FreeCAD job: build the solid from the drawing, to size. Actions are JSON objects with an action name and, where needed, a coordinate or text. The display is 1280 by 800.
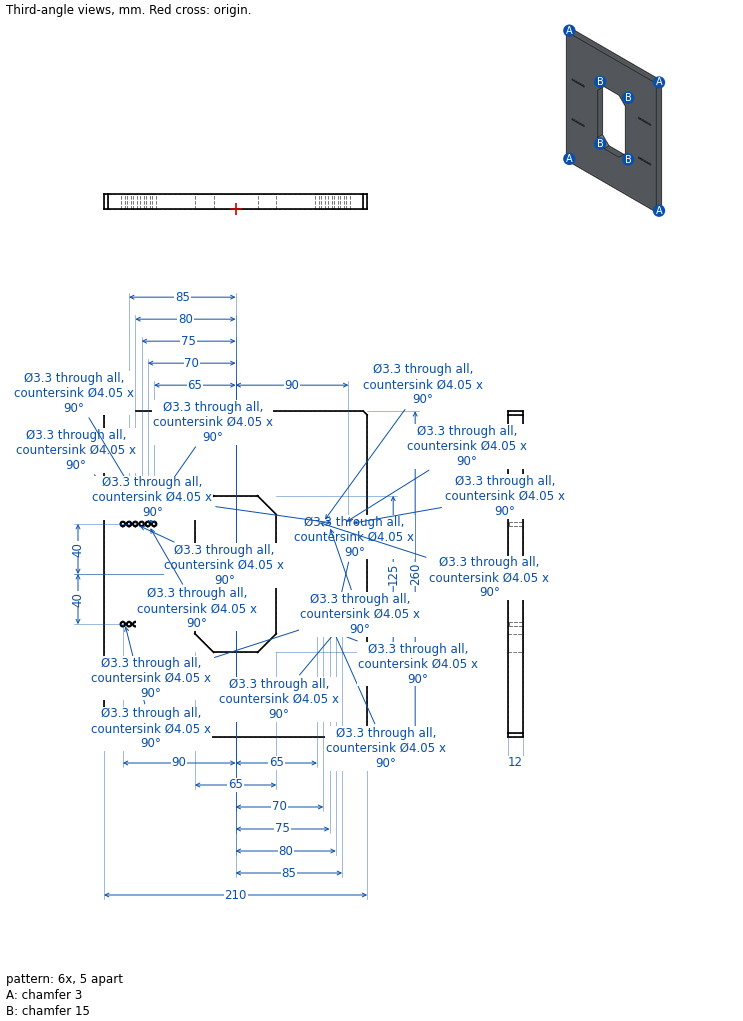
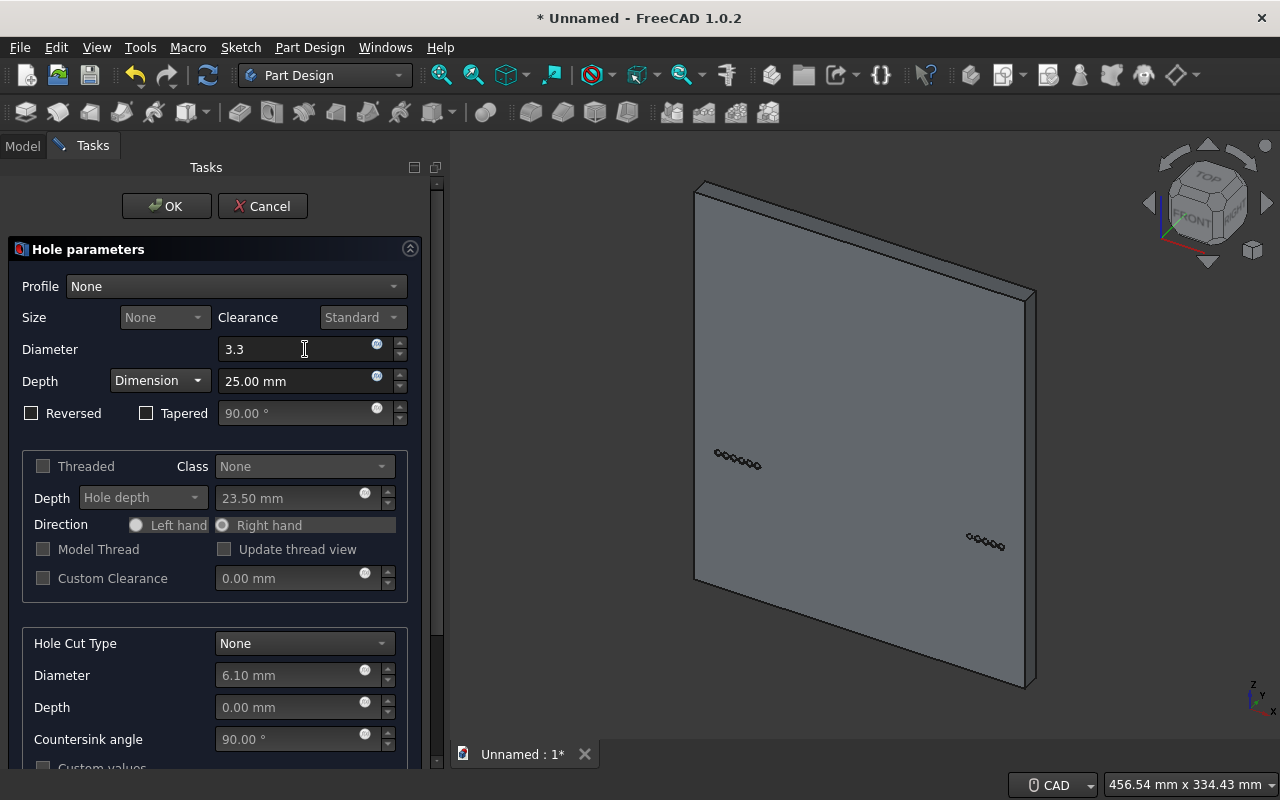
{"action": "left_click", "coordinate": [161, 380]}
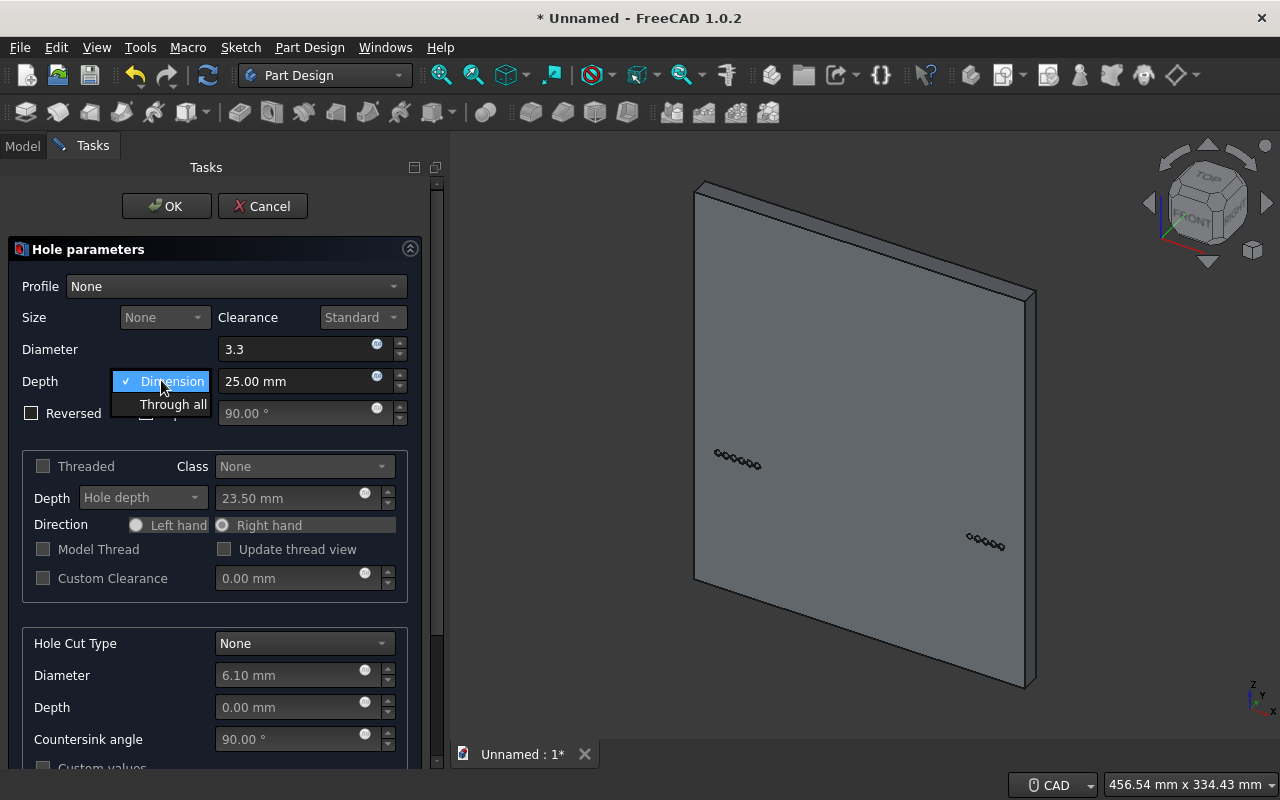
{"action": "left_click", "coordinate": [160, 404]}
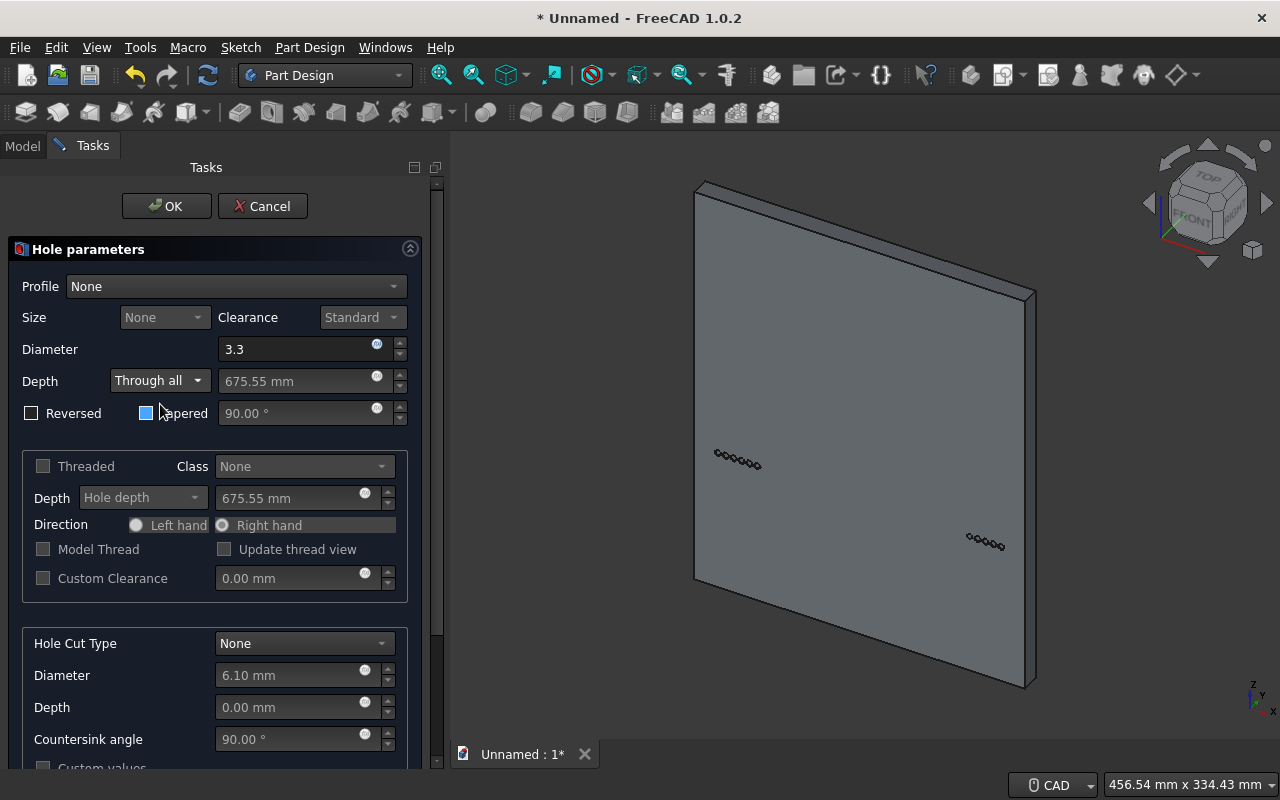
{"action": "left_click", "coordinate": [306, 644]}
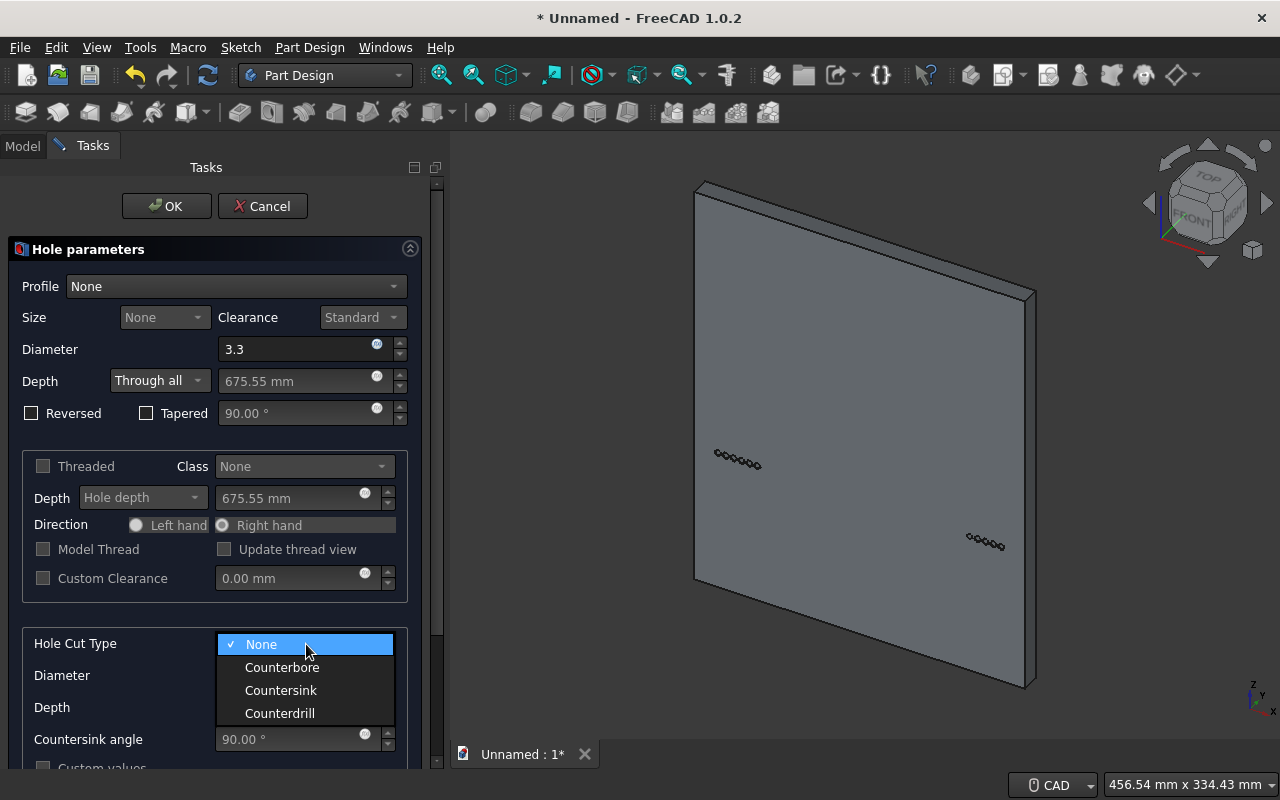
{"action": "left_click", "coordinate": [304, 690]}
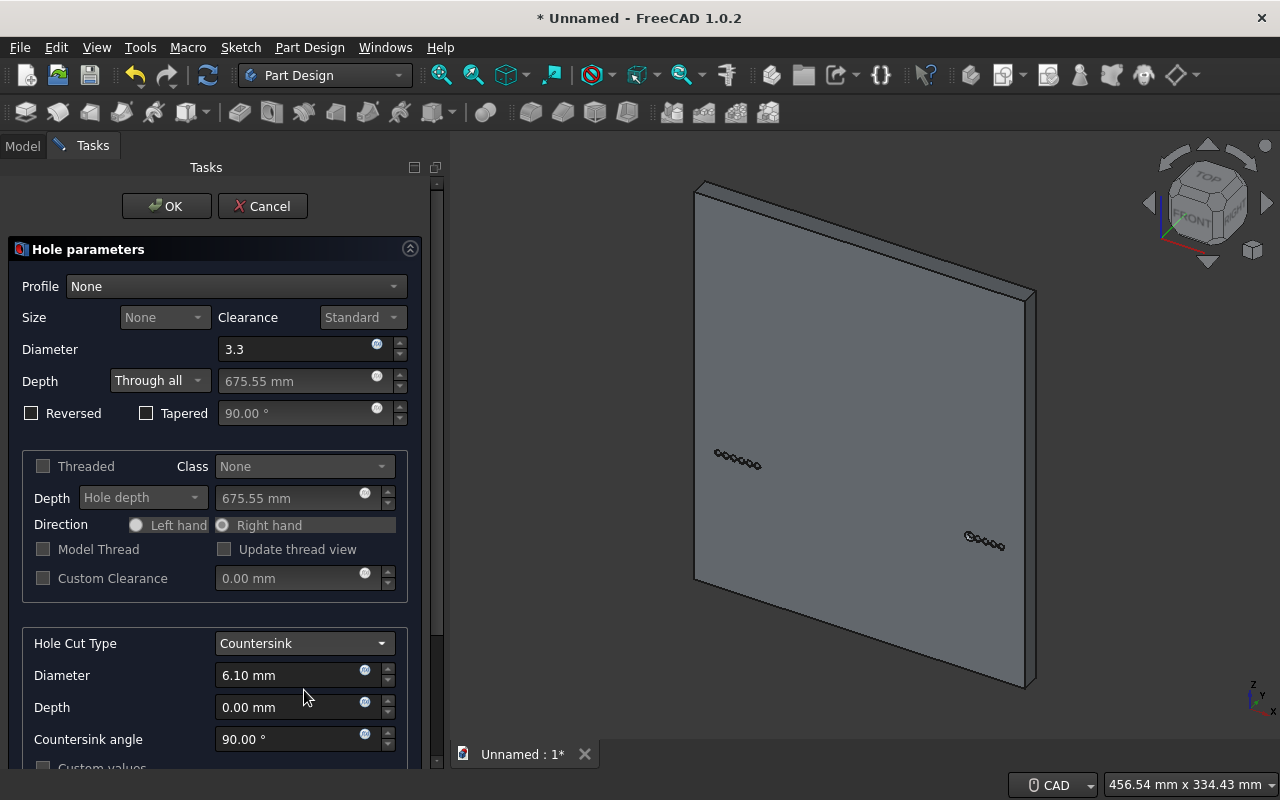
{"action": "triple_click", "coordinate": [298, 675]}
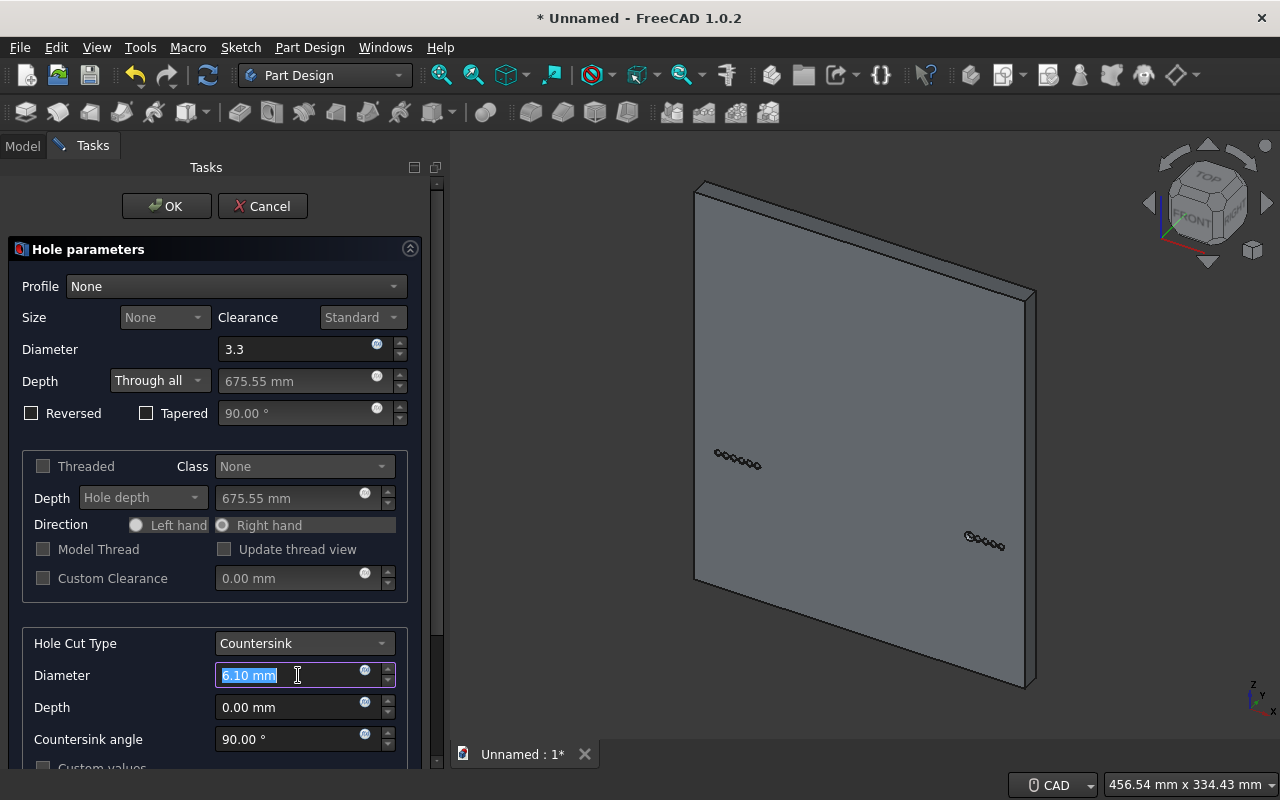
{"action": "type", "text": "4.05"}
{"action": "key", "text": "Tab"}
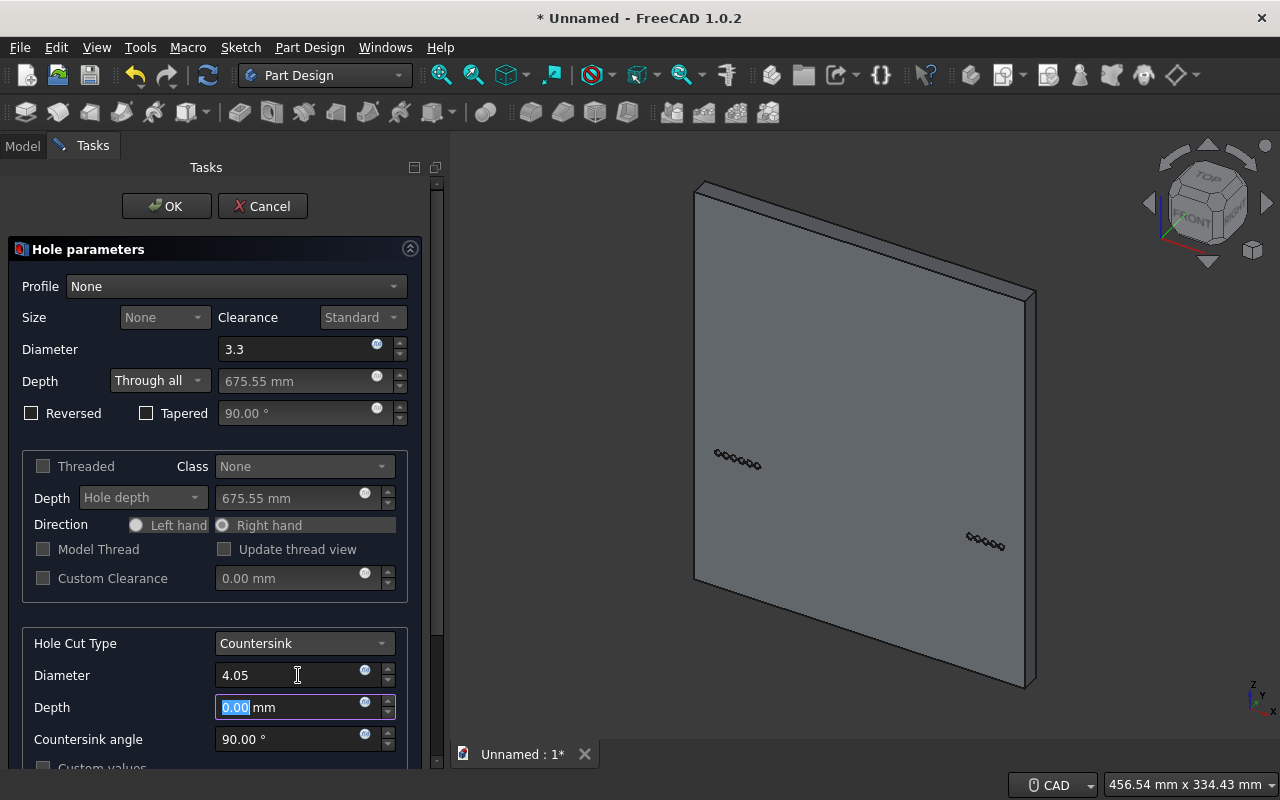
{"action": "left_click", "coordinate": [167, 206]}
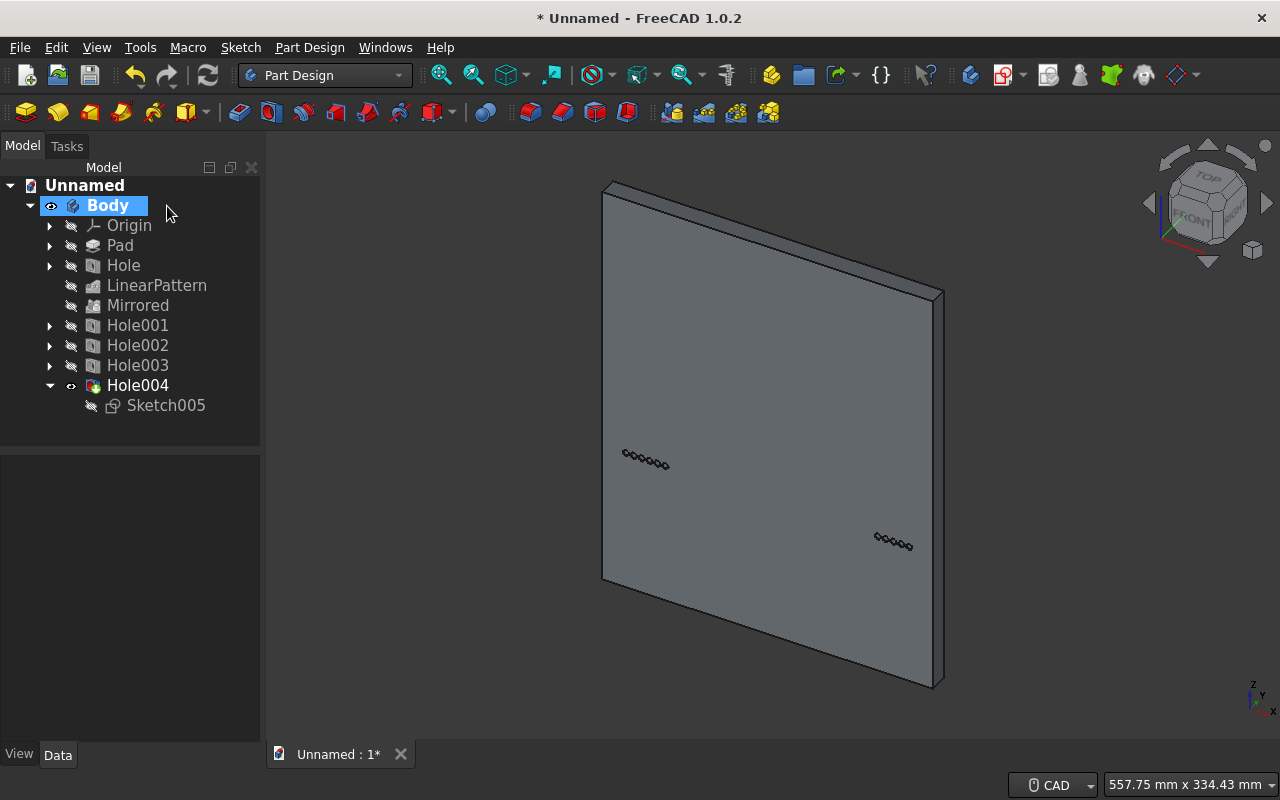
{"action": "left_click", "coordinate": [1004, 76]}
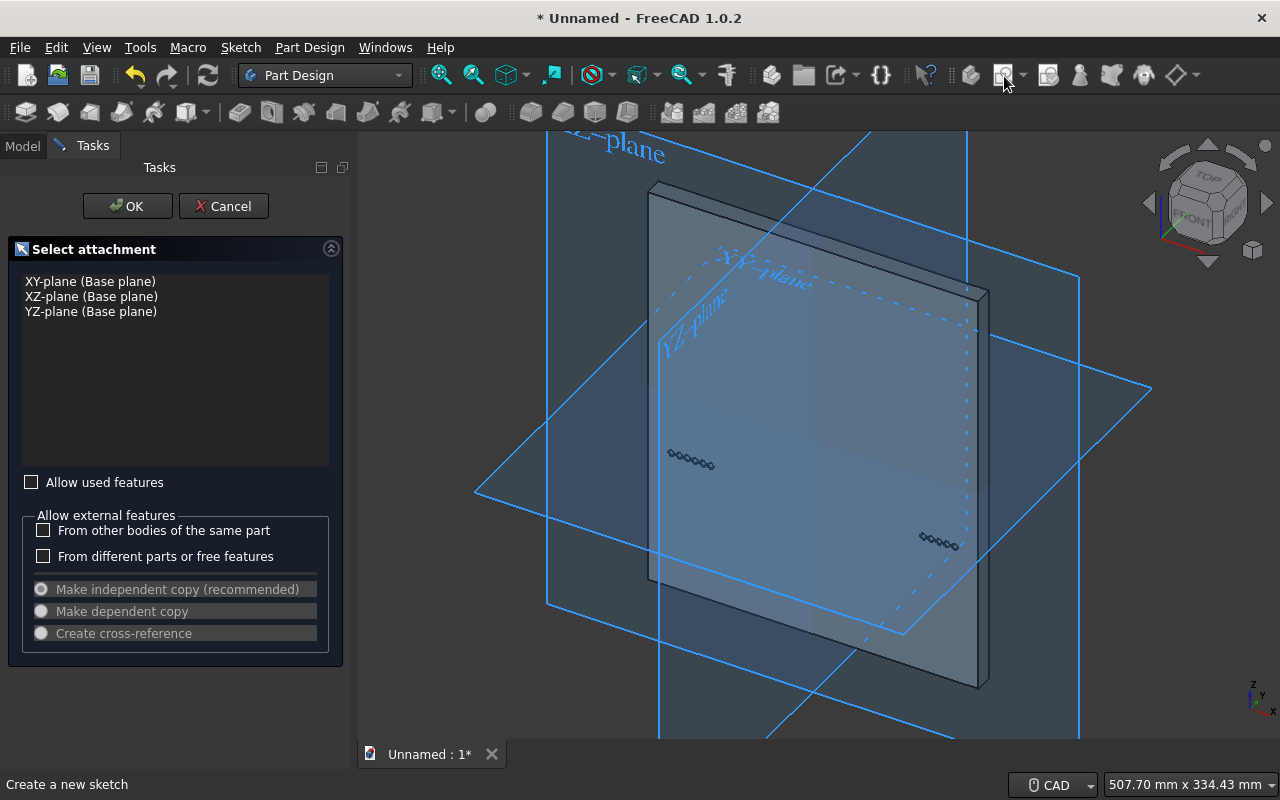
{"action": "left_click", "coordinate": [82, 296]}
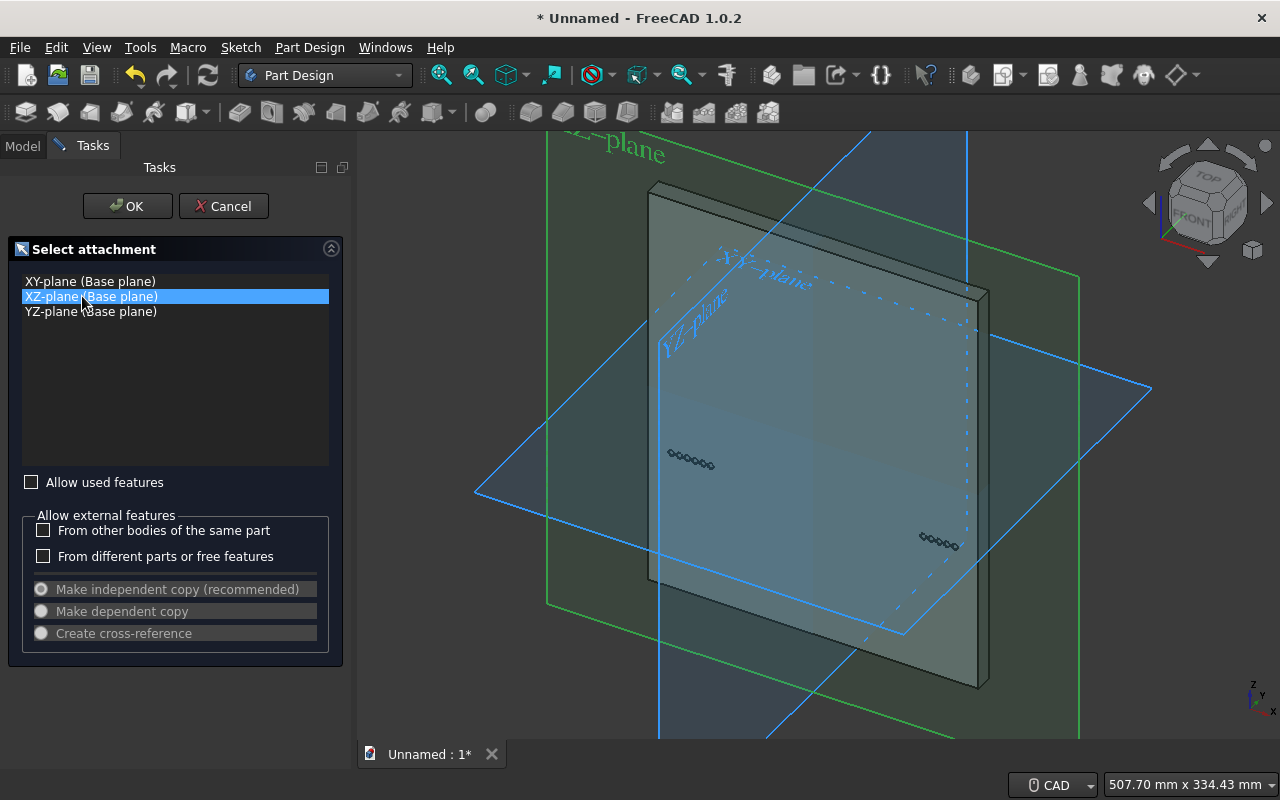
{"action": "left_click", "coordinate": [128, 206]}